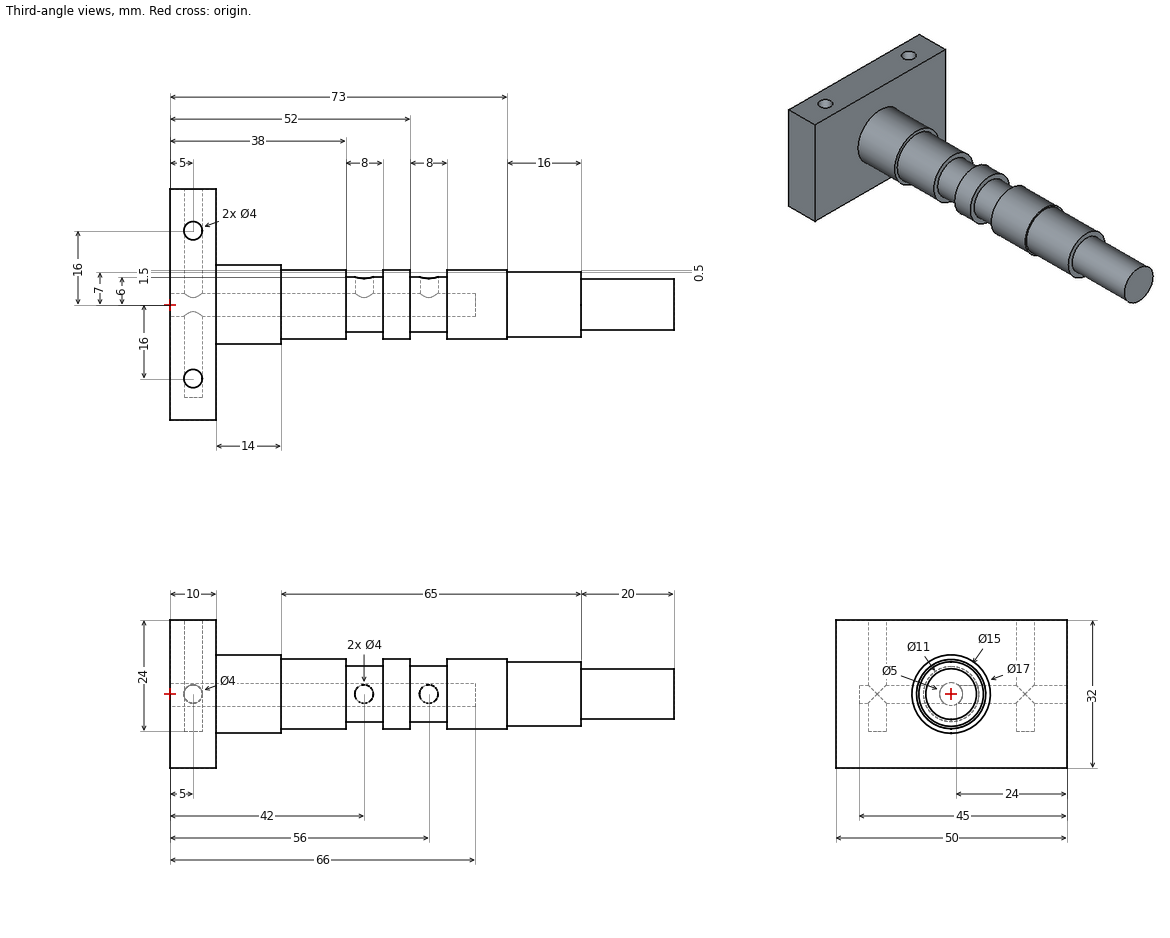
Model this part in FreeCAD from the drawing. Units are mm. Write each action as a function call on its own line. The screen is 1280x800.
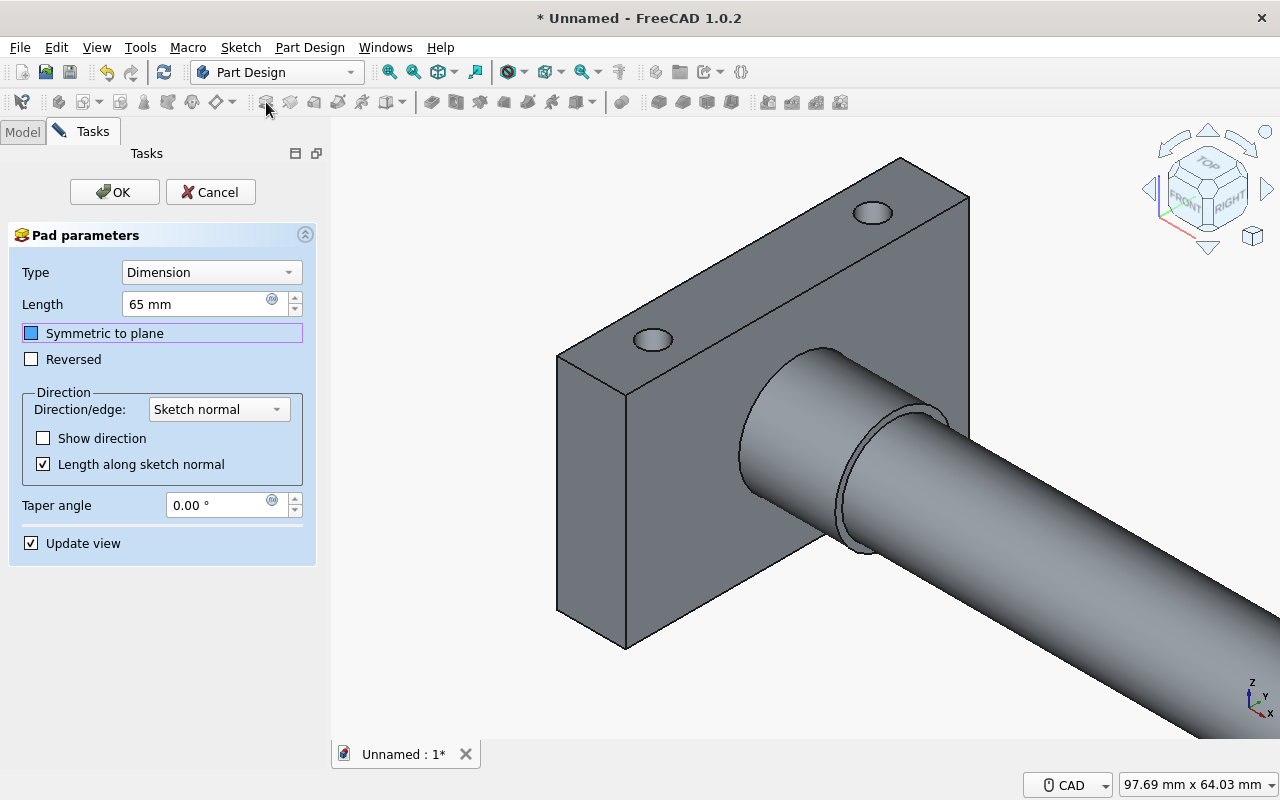
click(115, 192)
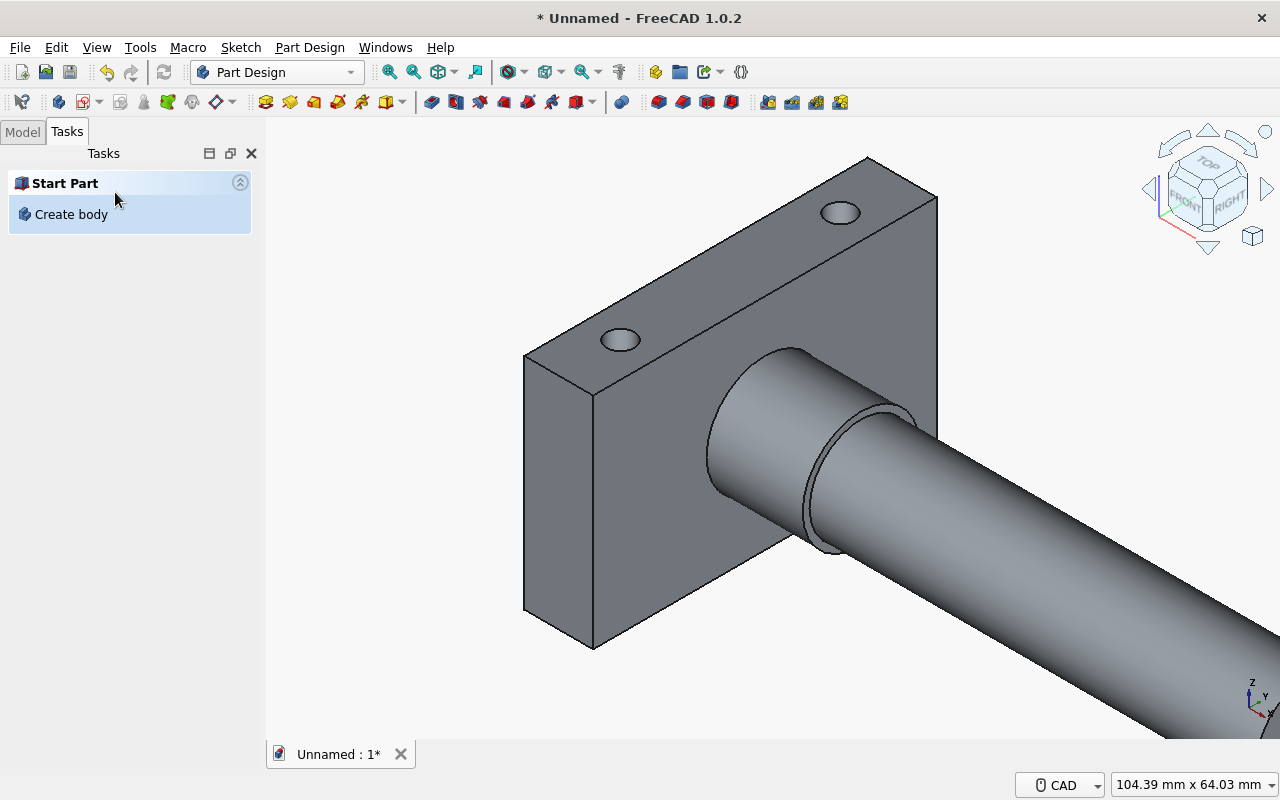
click(390, 72)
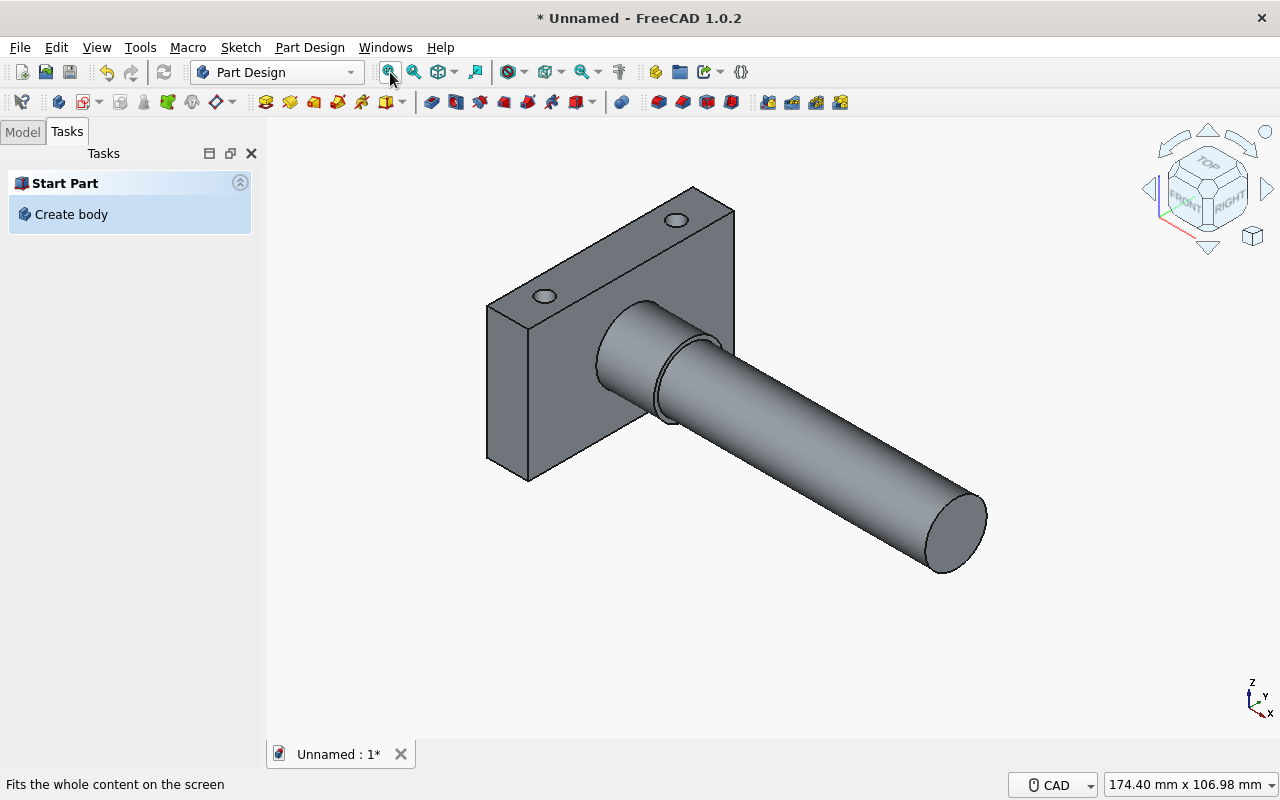
click(84, 102)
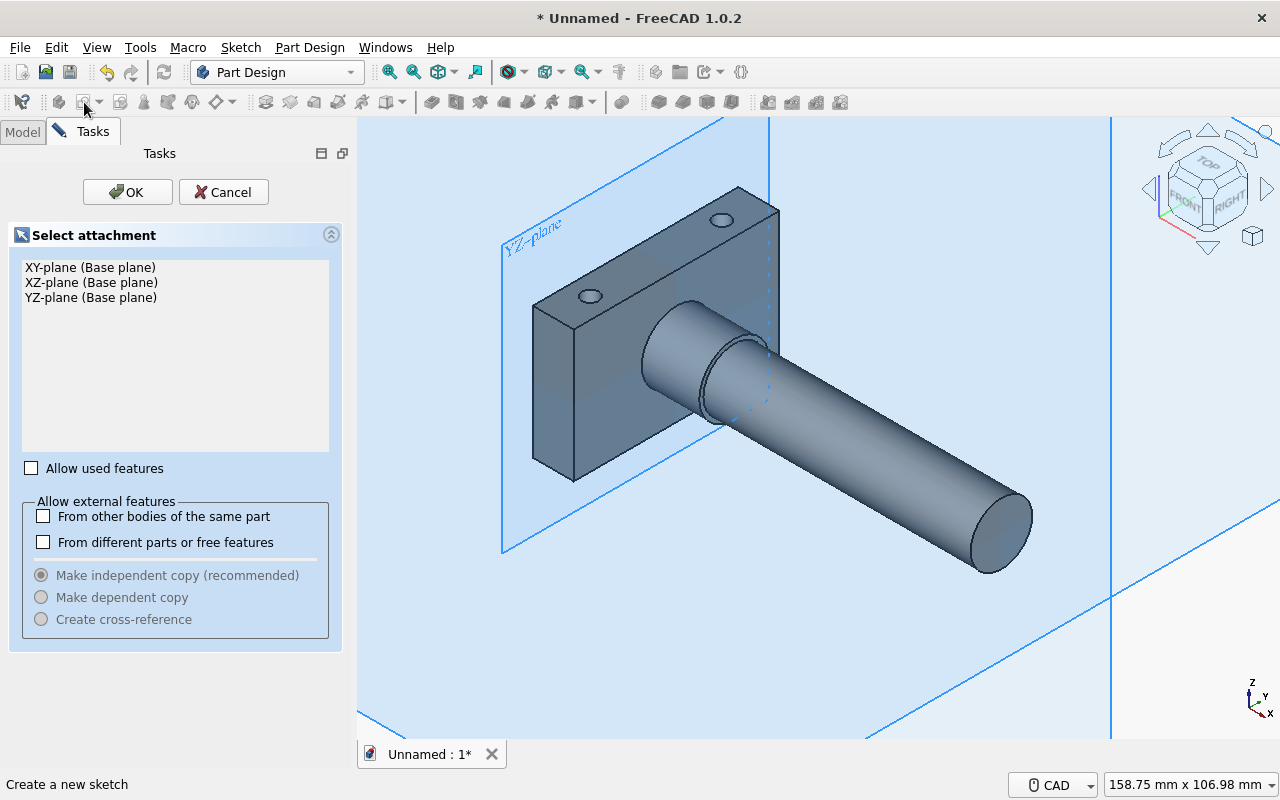
click(82, 268)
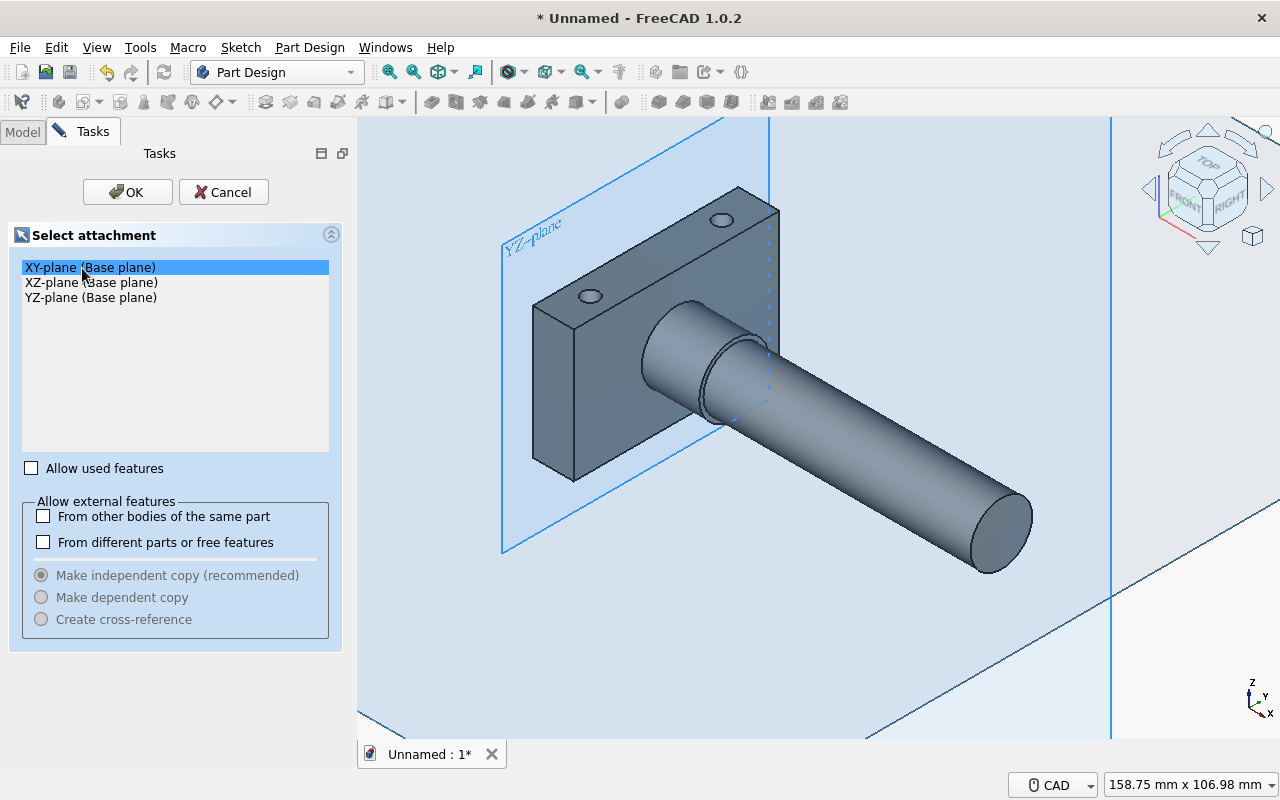
click(128, 192)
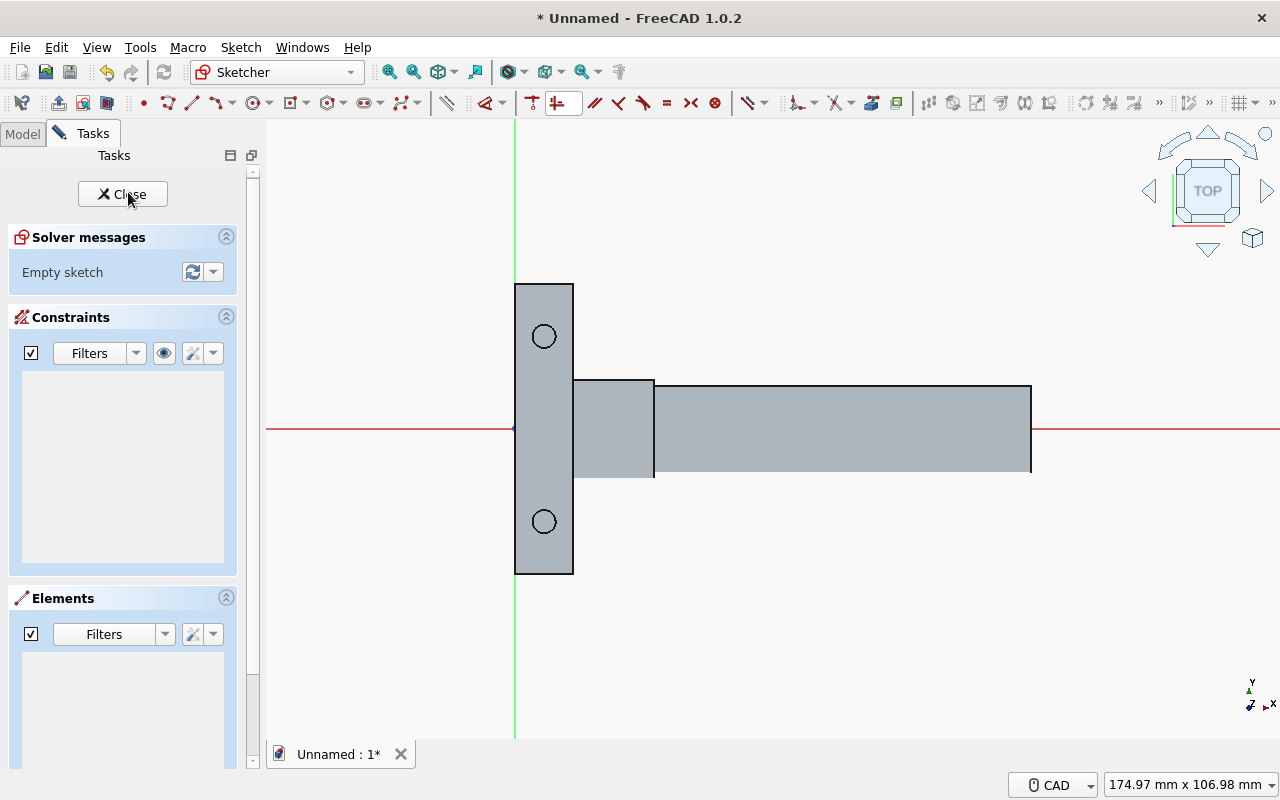
click(108, 104)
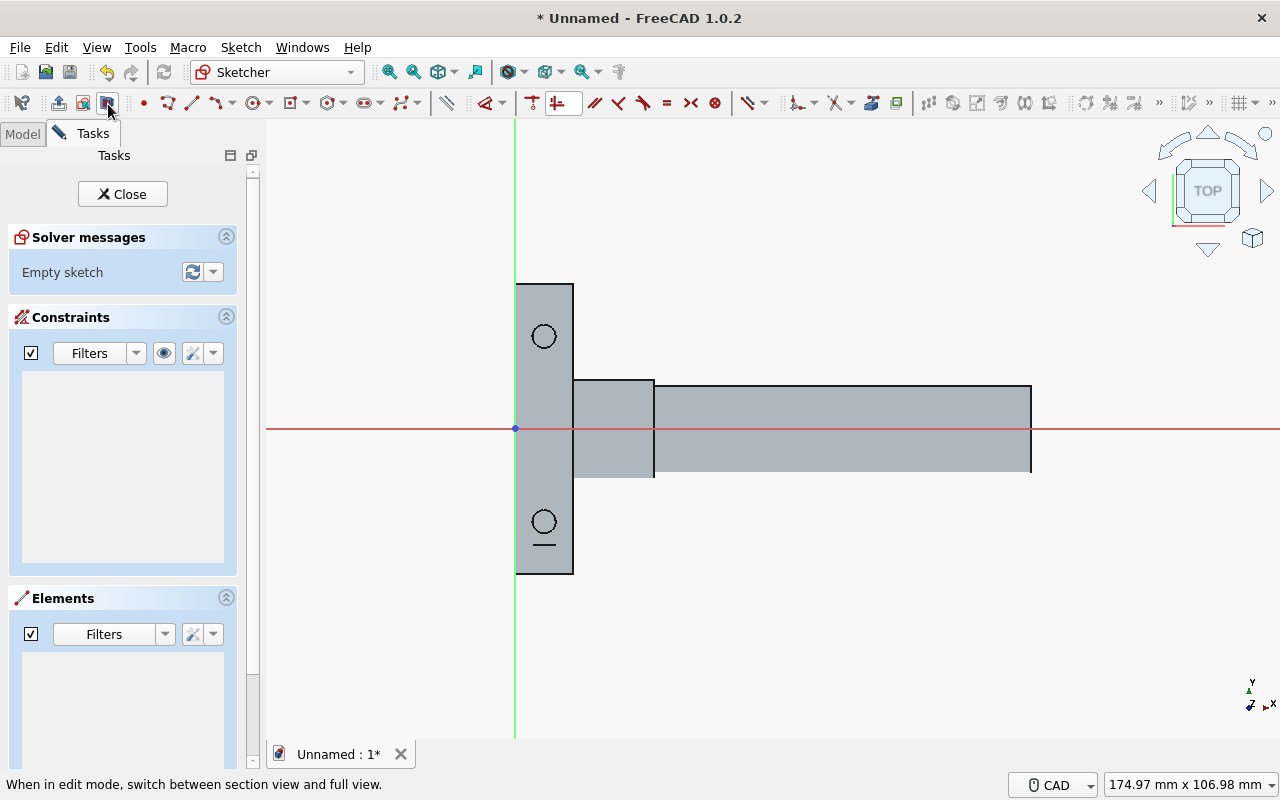
scroll(823, 380, up, 8)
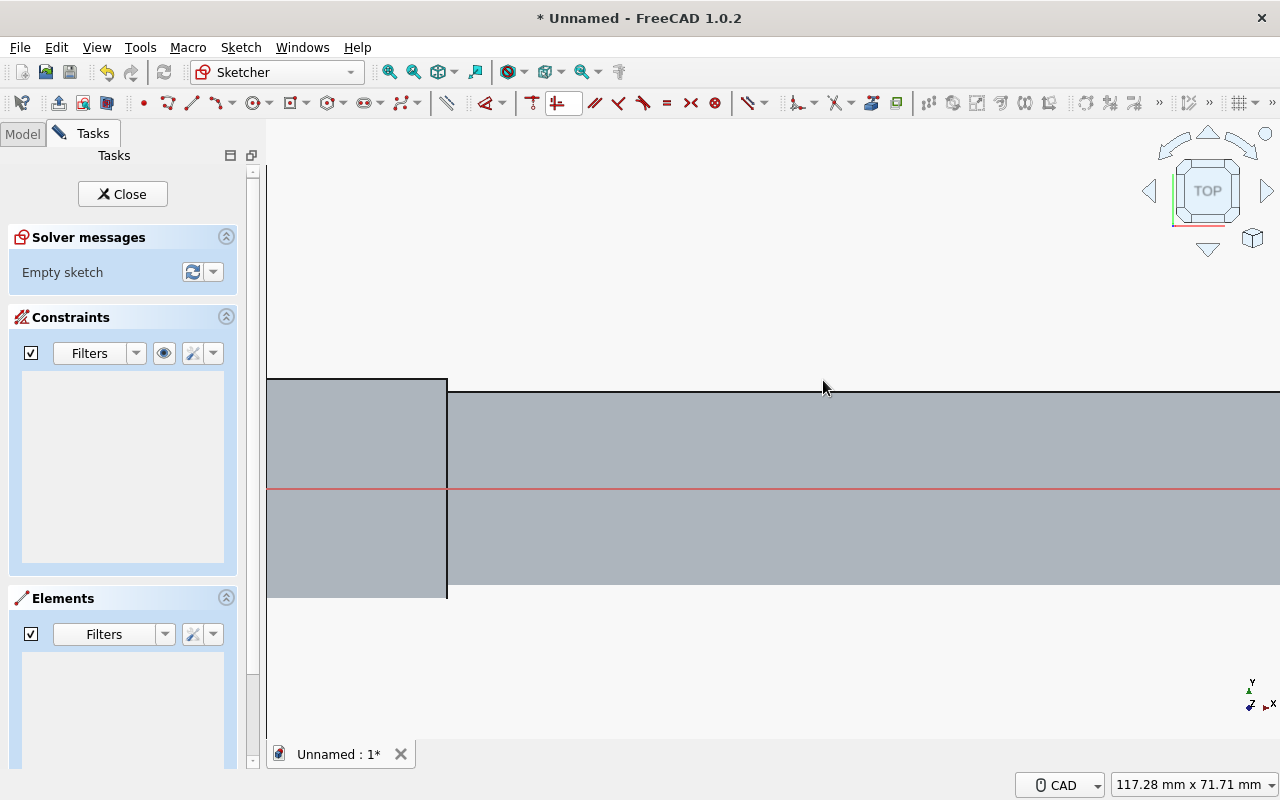
click(308, 104)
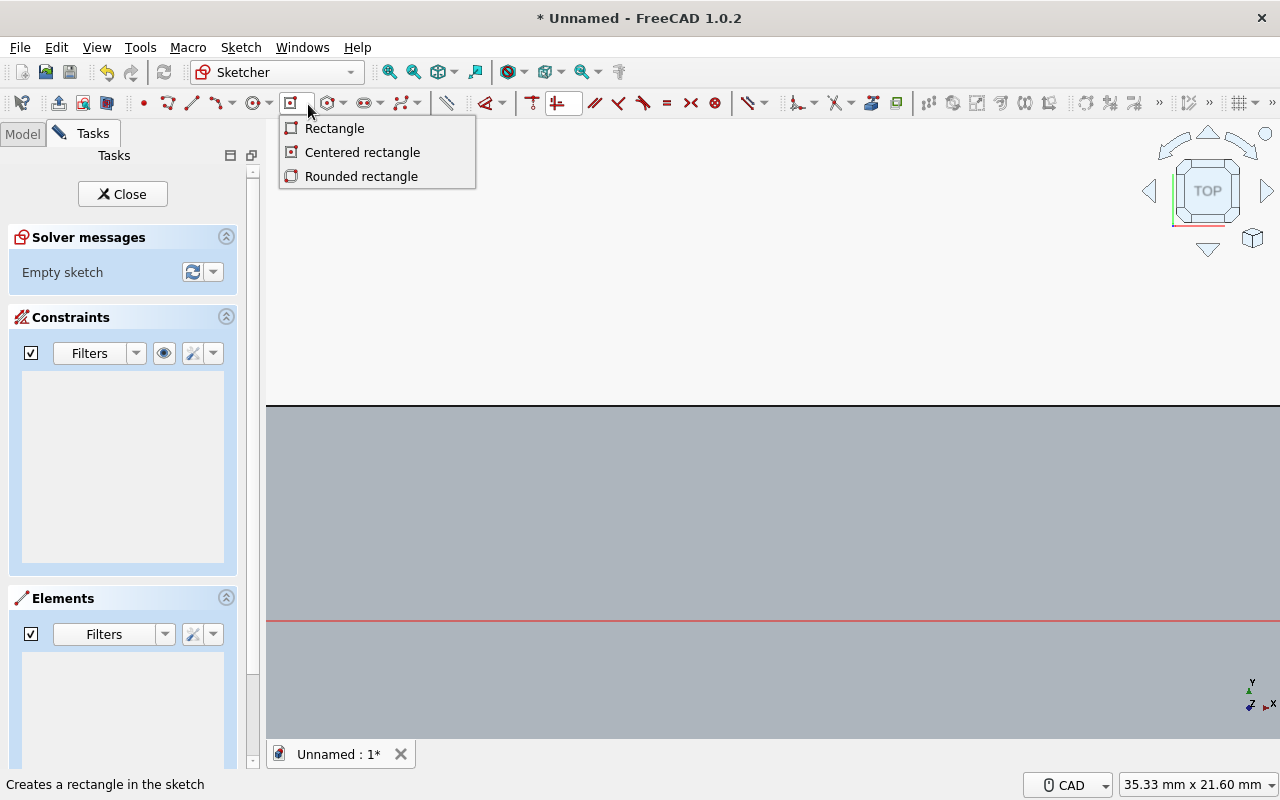
click(378, 128)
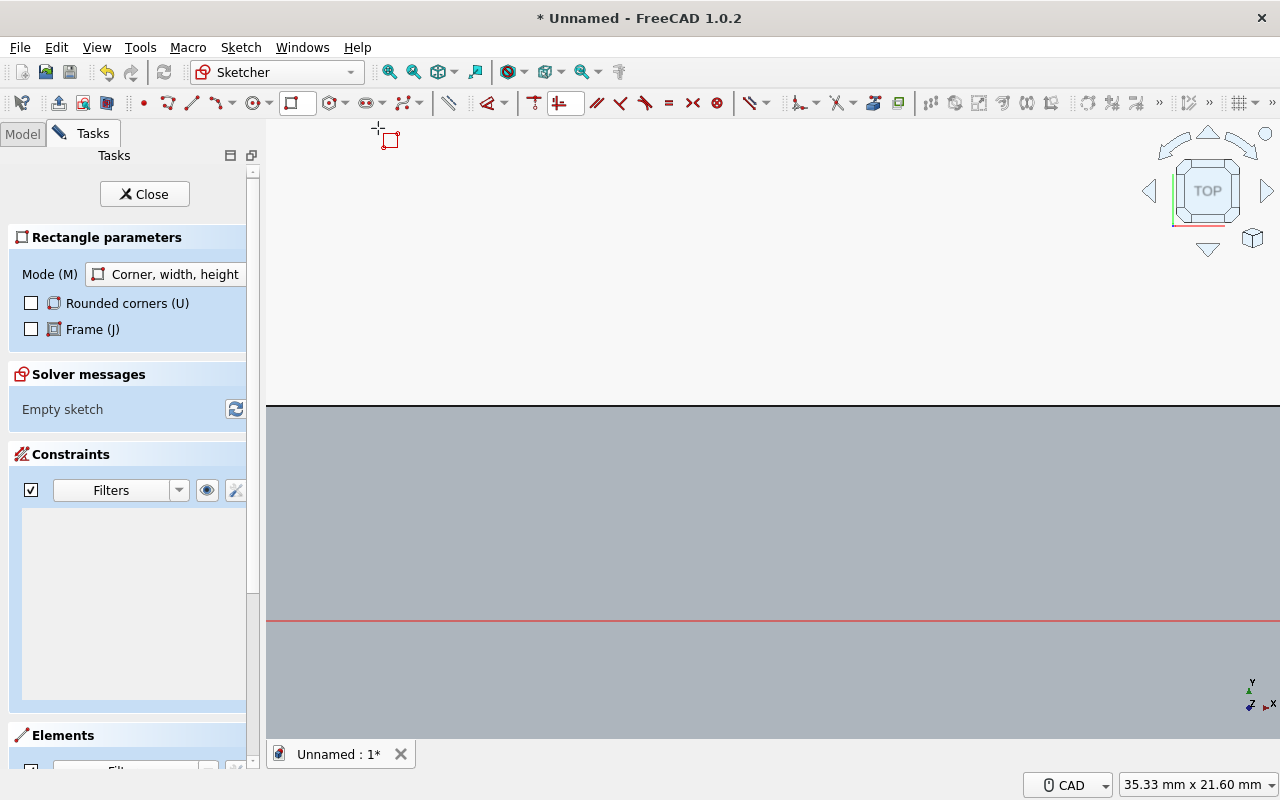
click(387, 406)
move(616, 449)